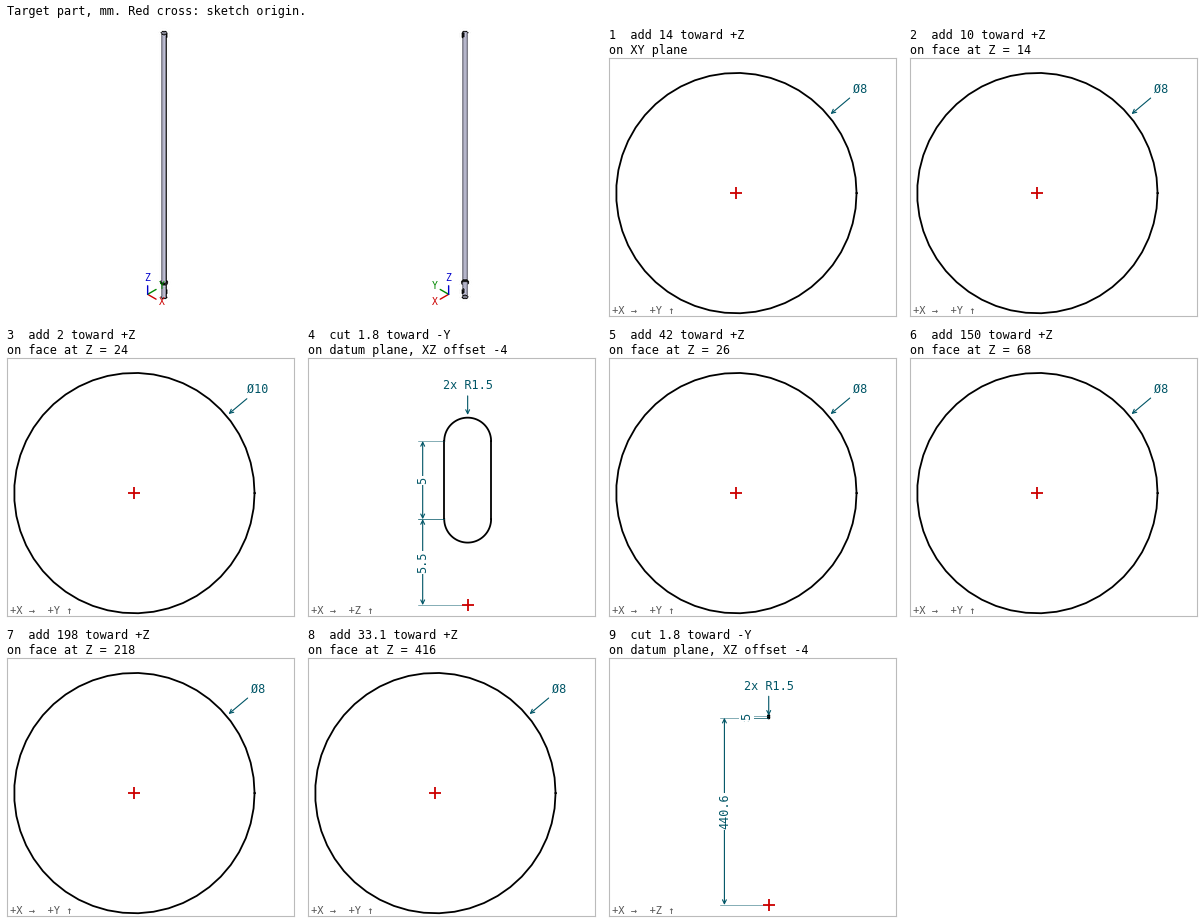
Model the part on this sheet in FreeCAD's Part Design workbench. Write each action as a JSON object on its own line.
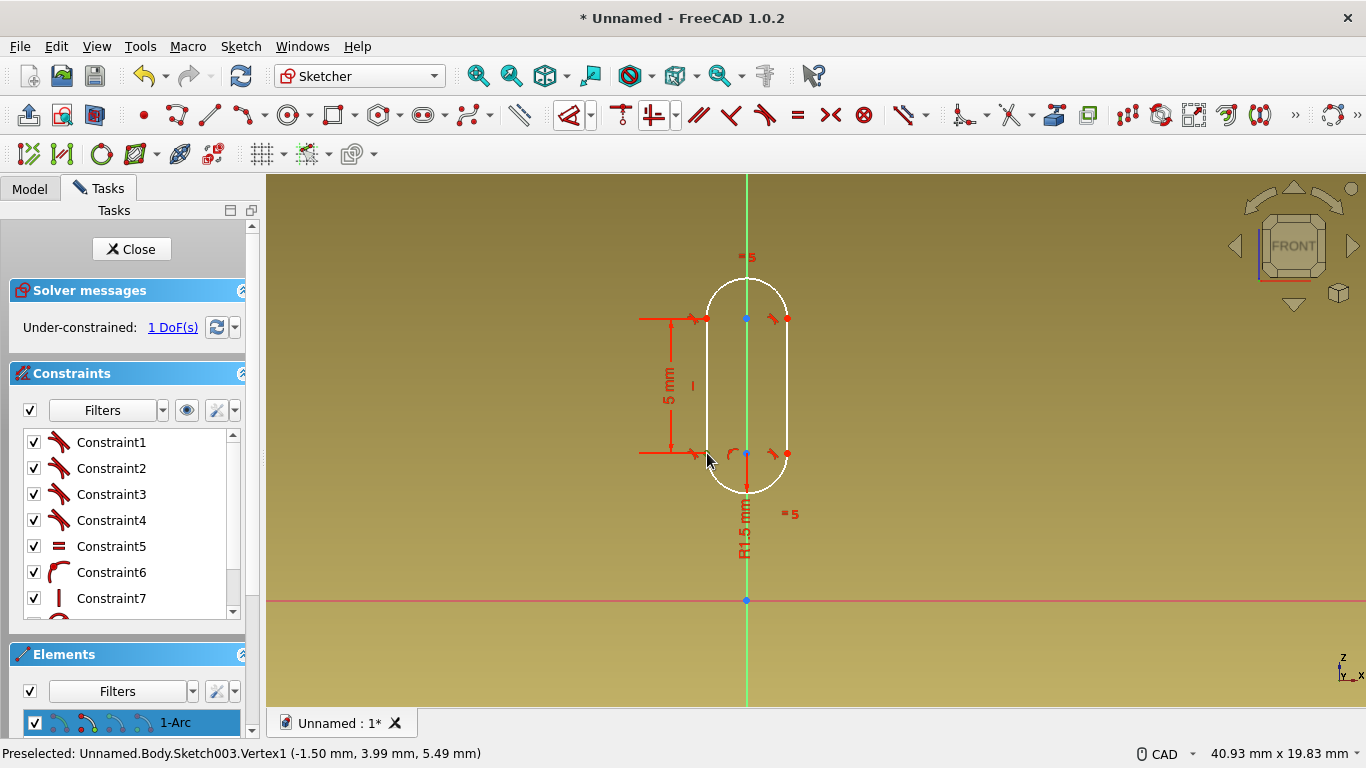
{"action": "key", "text": "i"}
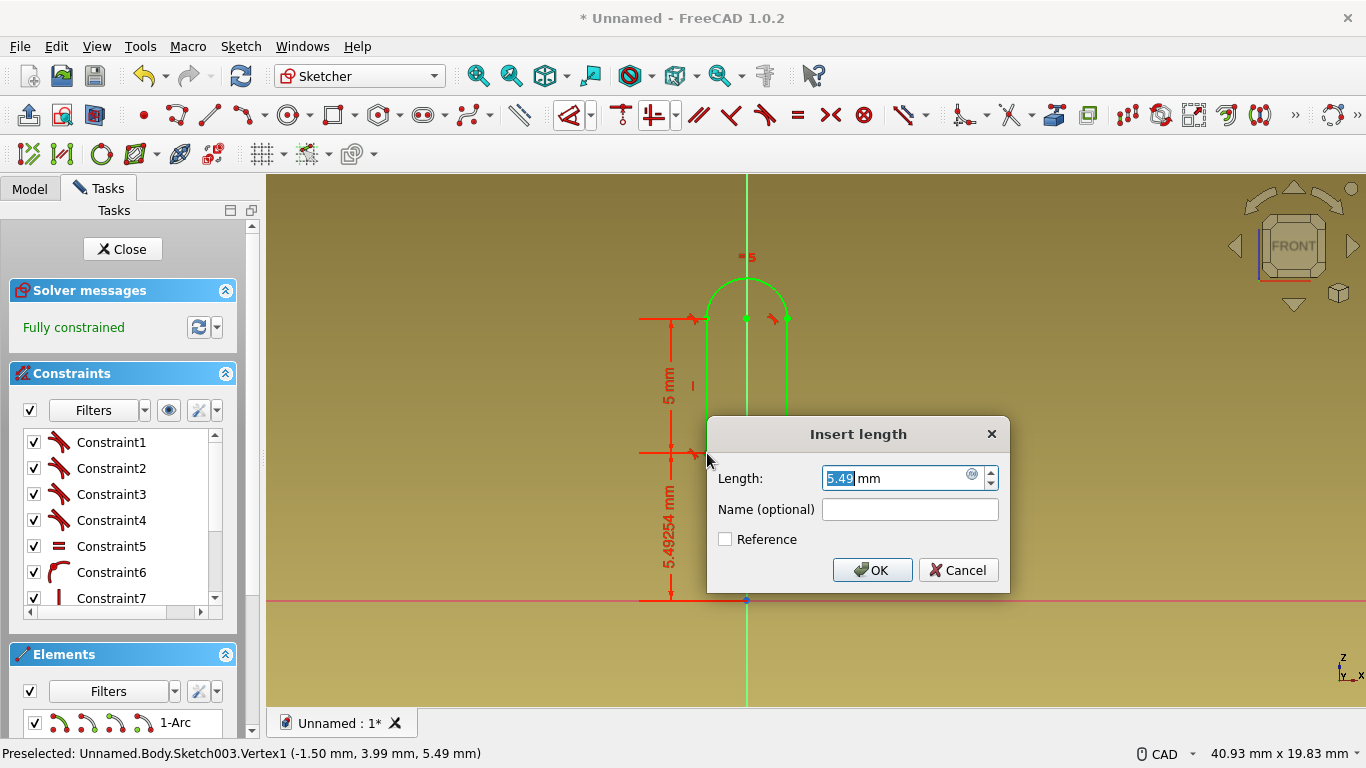
{"action": "type", "text": "5.5"}
{"action": "key", "text": "Return"}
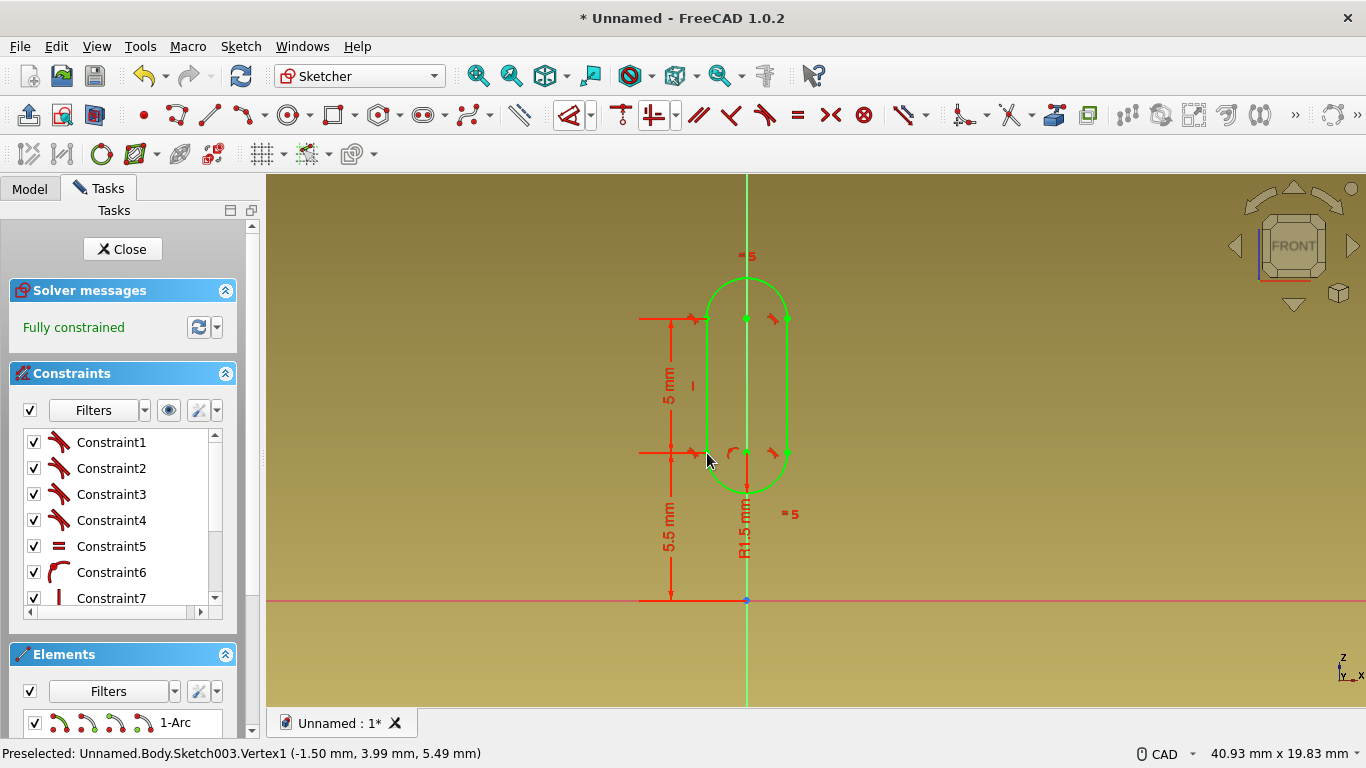
{"action": "left_click", "coordinate": [123, 249]}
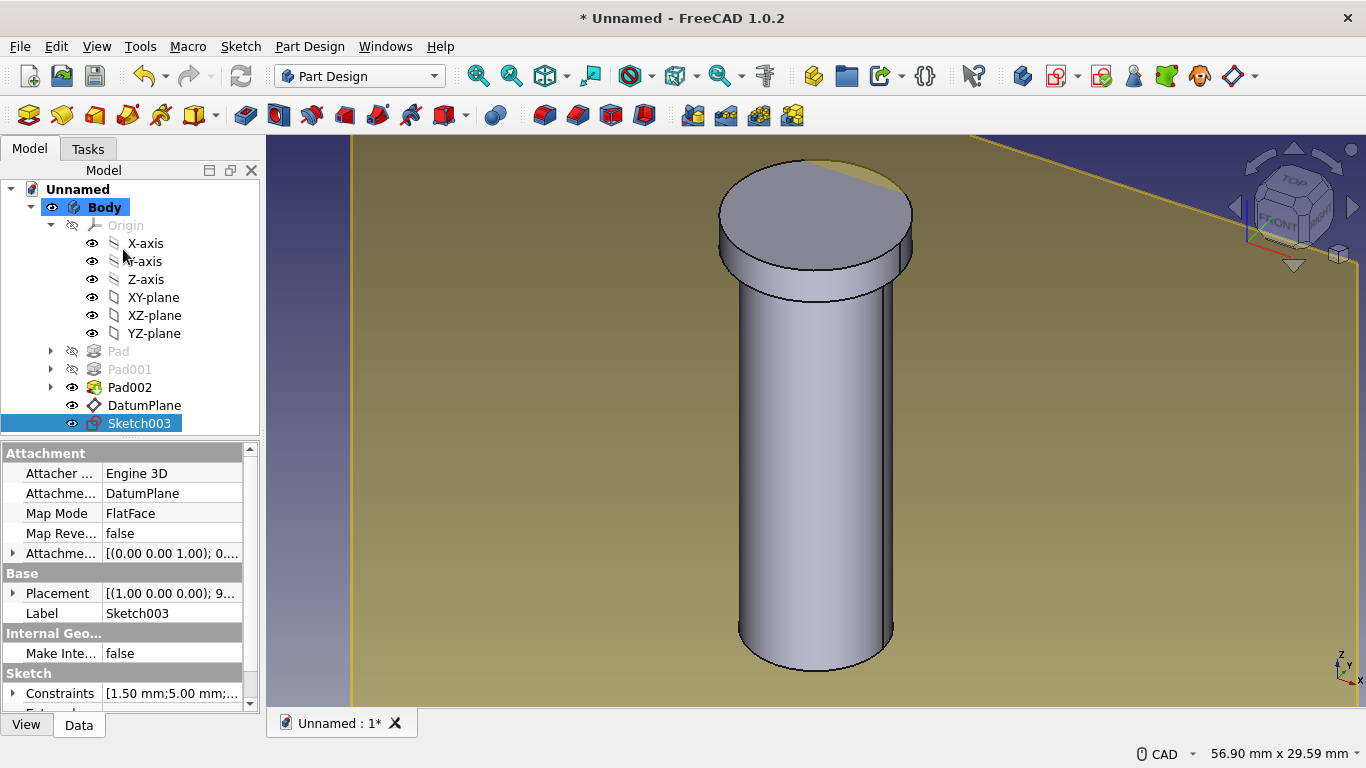
{"action": "left_click", "coordinate": [246, 116]}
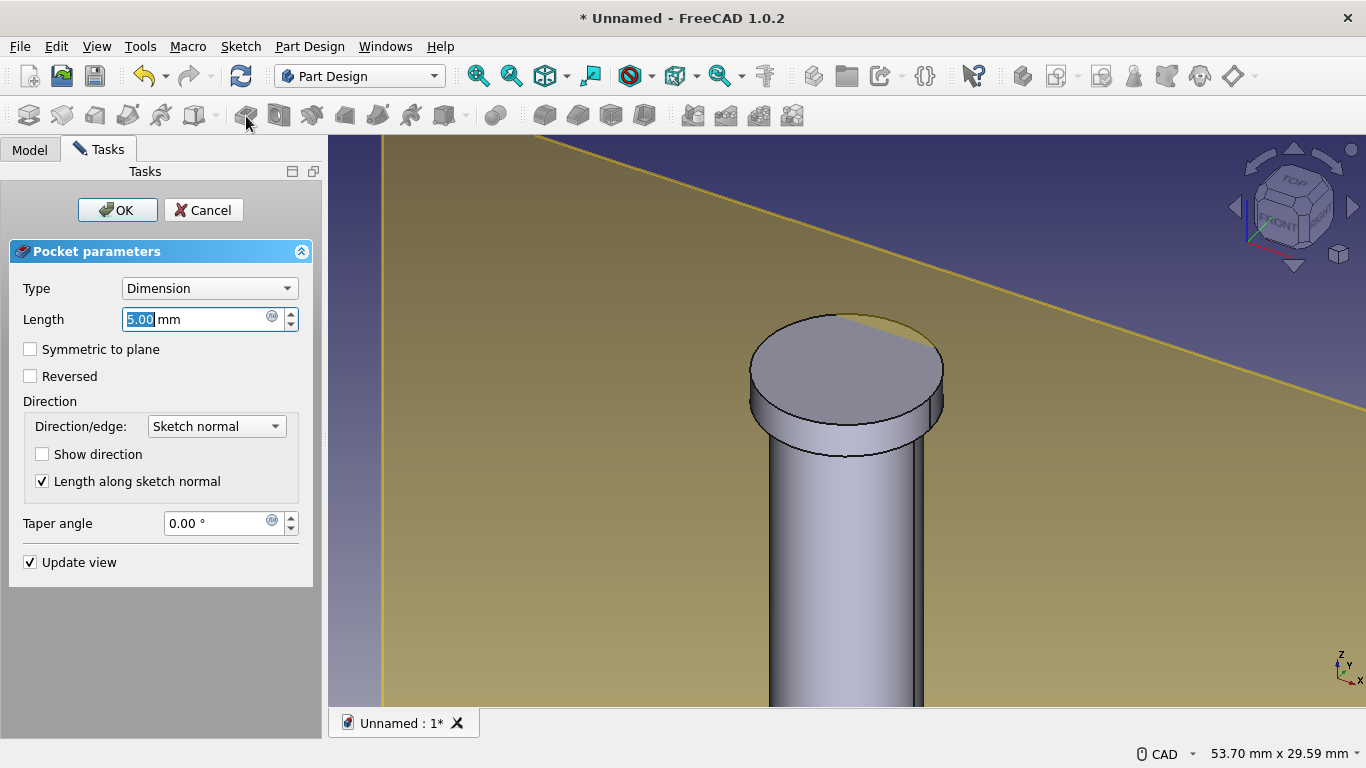
{"action": "type", "text": "1.8"}
{"action": "key", "text": "Tab"}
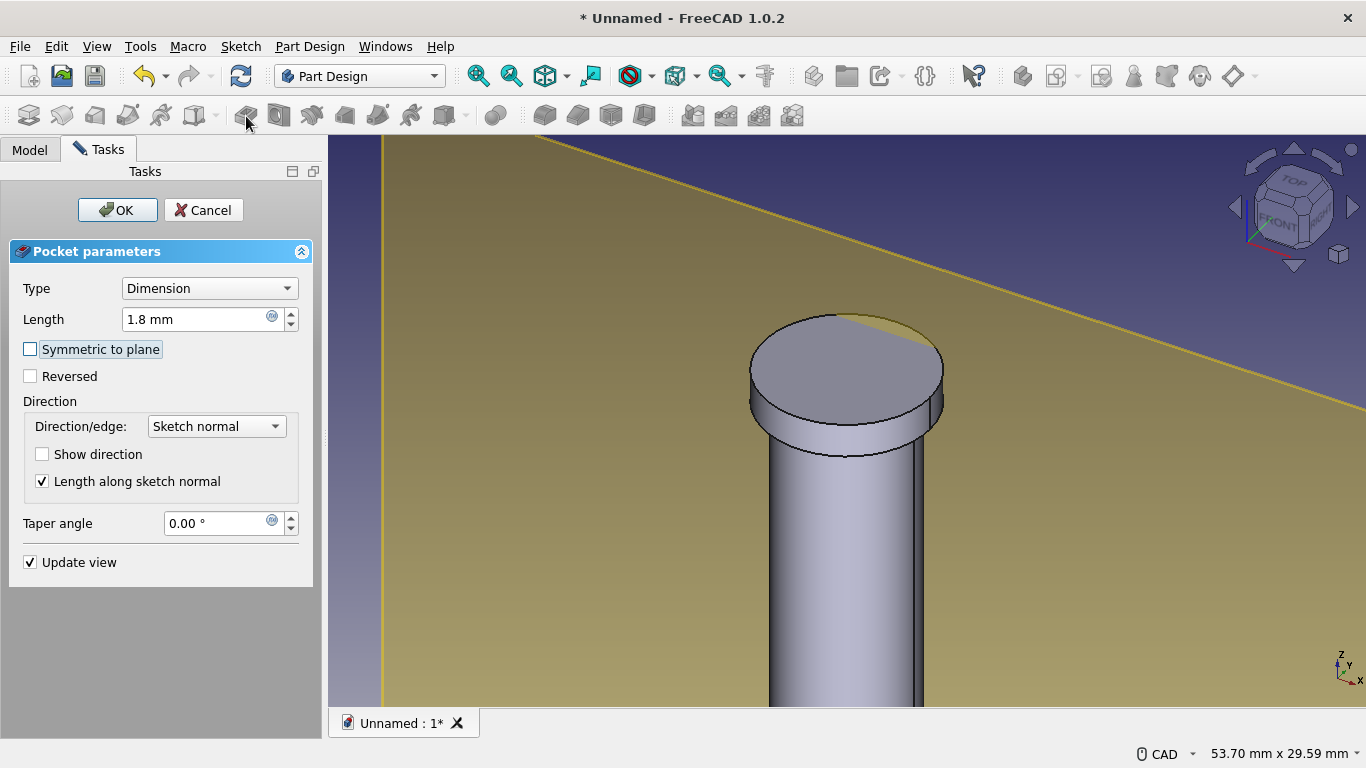
{"action": "left_click", "coordinate": [31, 376]}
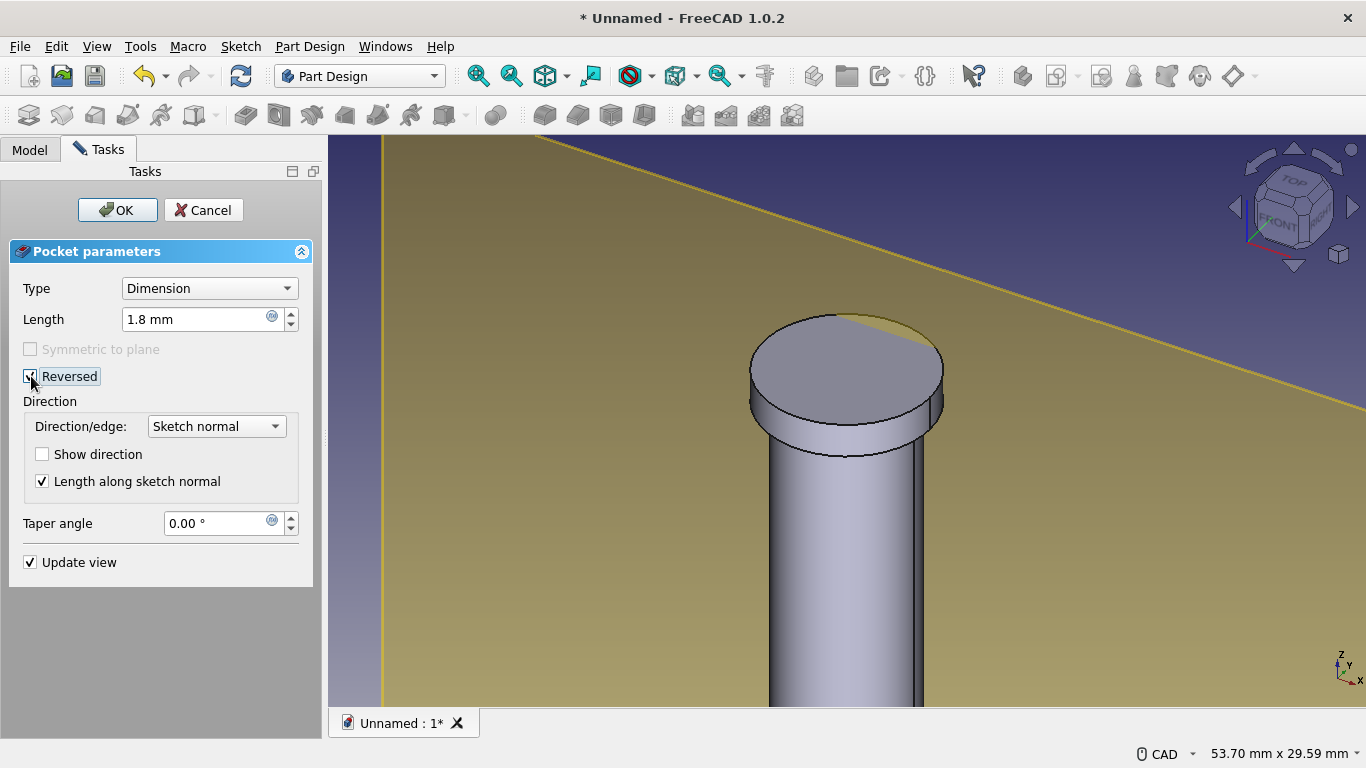
{"action": "left_click", "coordinate": [118, 210]}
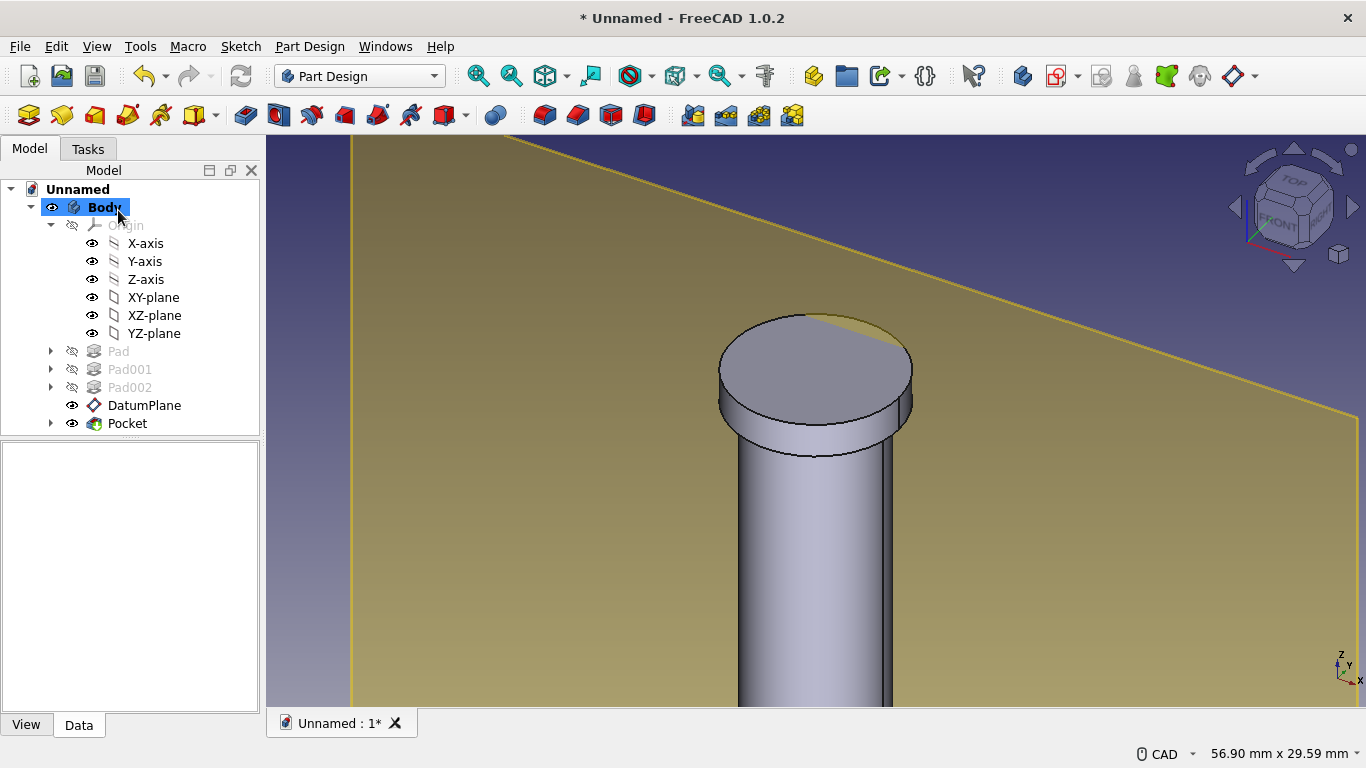
{"action": "left_click", "coordinate": [117, 405]}
{"action": "key", "text": "space"}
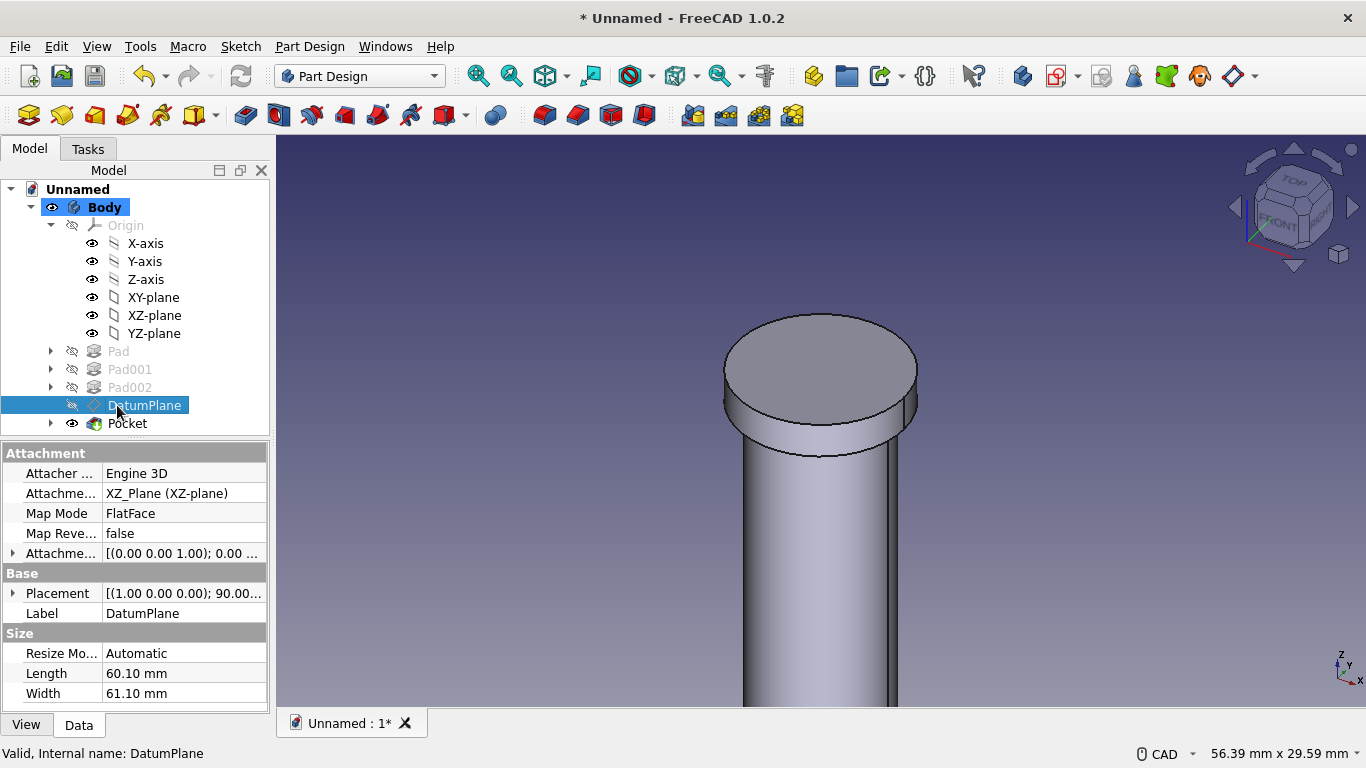
{"action": "left_click", "coordinate": [479, 76]}